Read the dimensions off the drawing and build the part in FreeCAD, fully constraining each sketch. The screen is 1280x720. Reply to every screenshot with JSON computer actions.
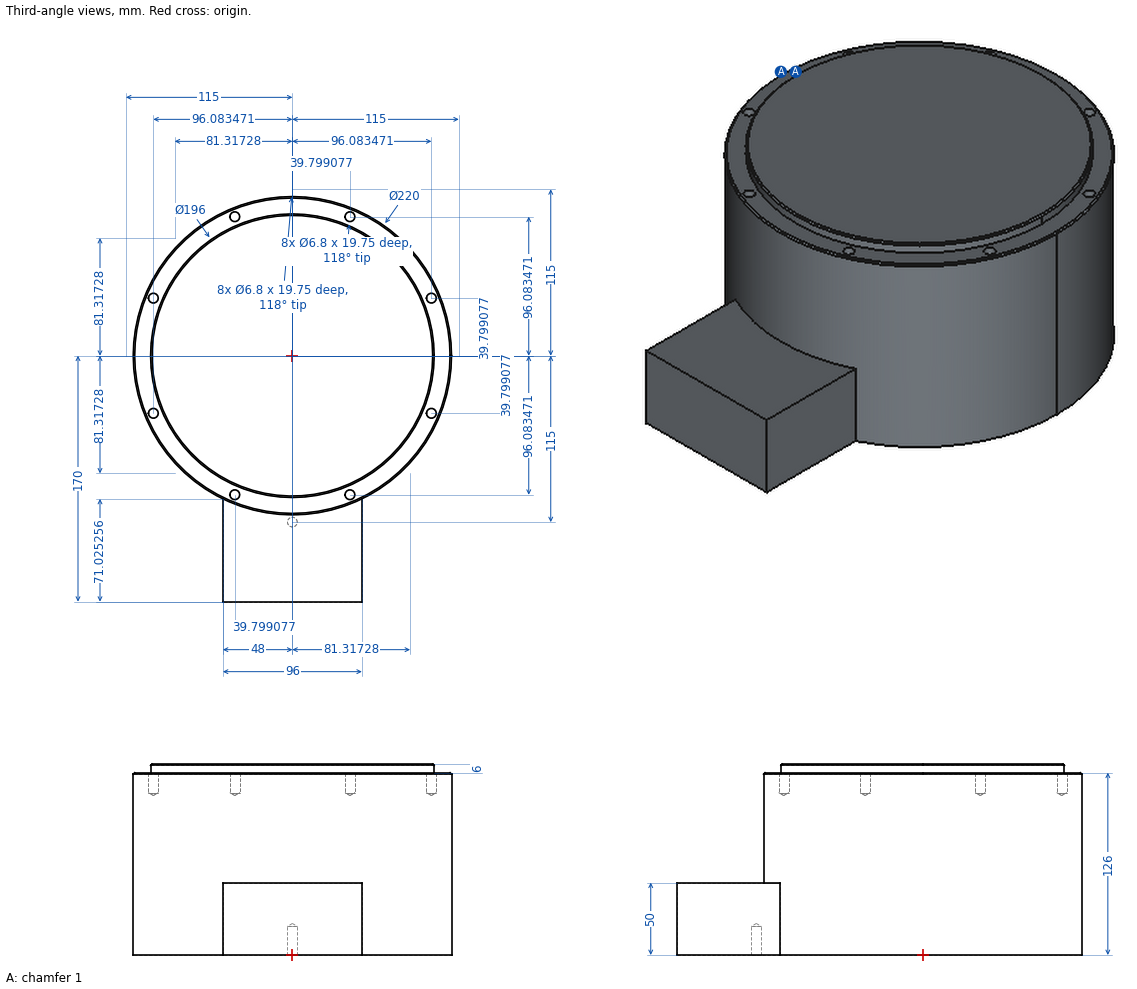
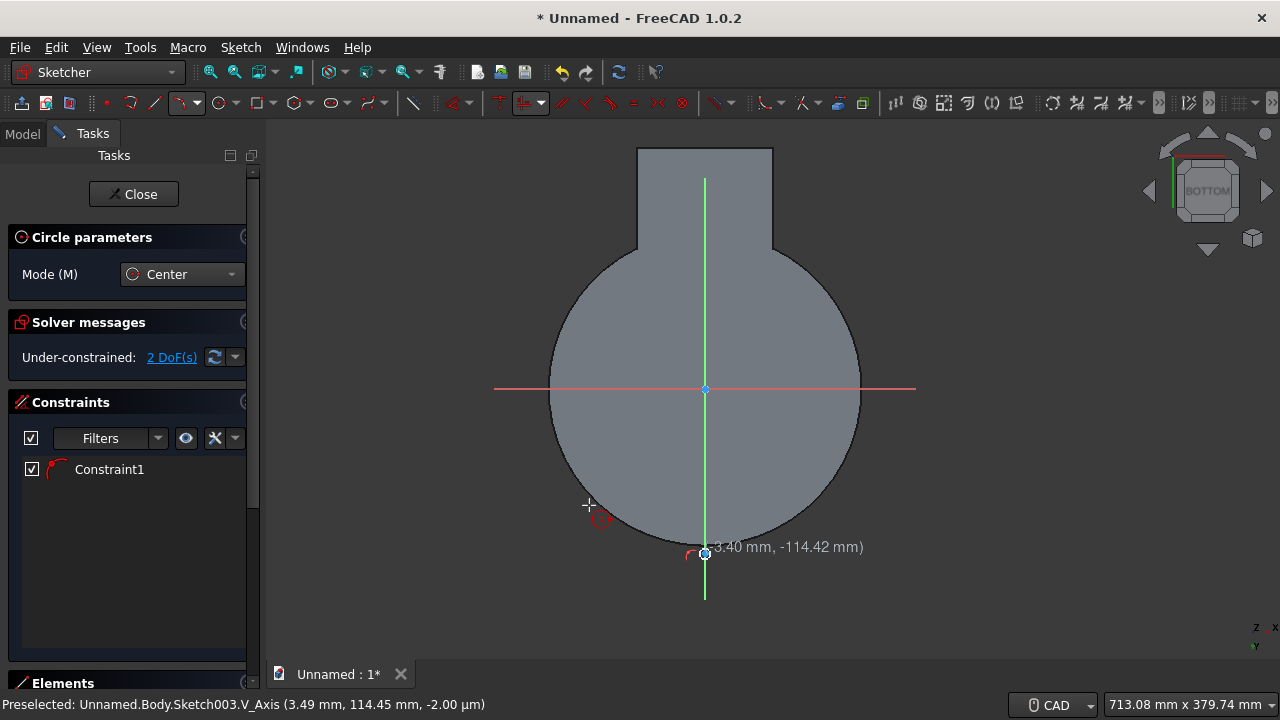
{"action": "left_click", "coordinate": [589, 505]}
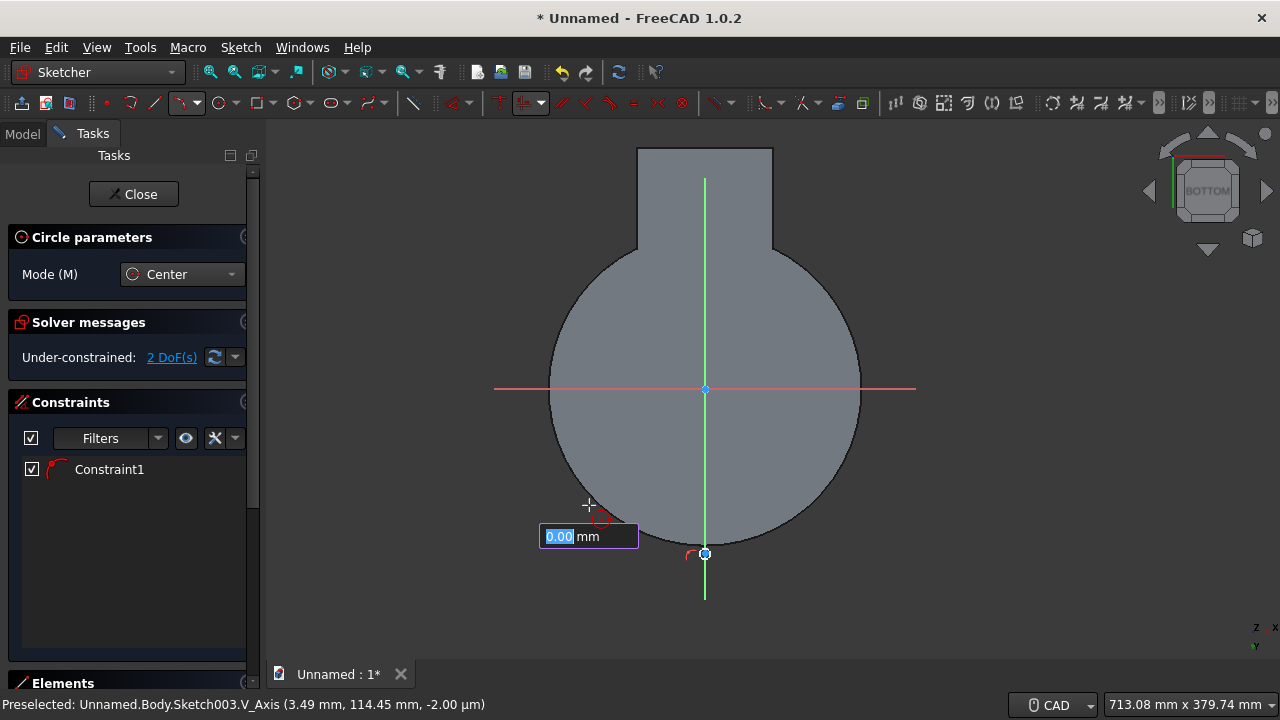
{"action": "scroll", "coordinate": [593, 502], "scroll_direction": "up", "scroll_amount": 6}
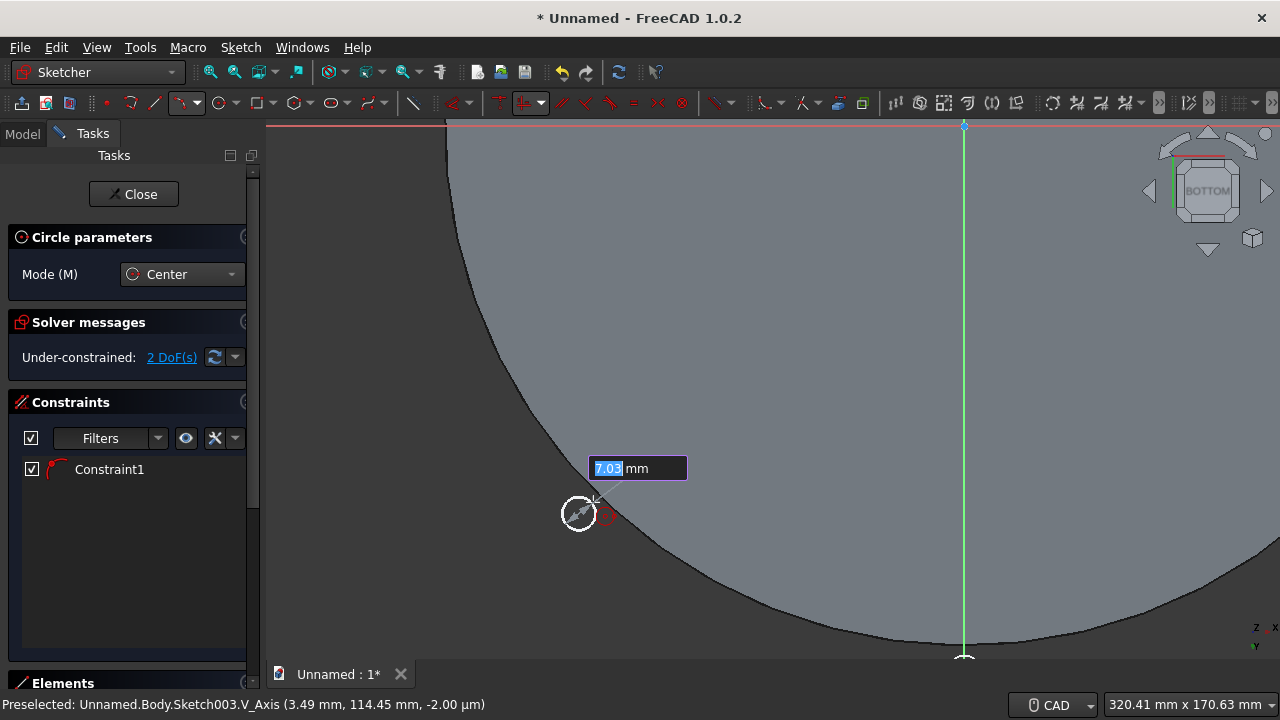
{"action": "left_click", "coordinate": [592, 499]}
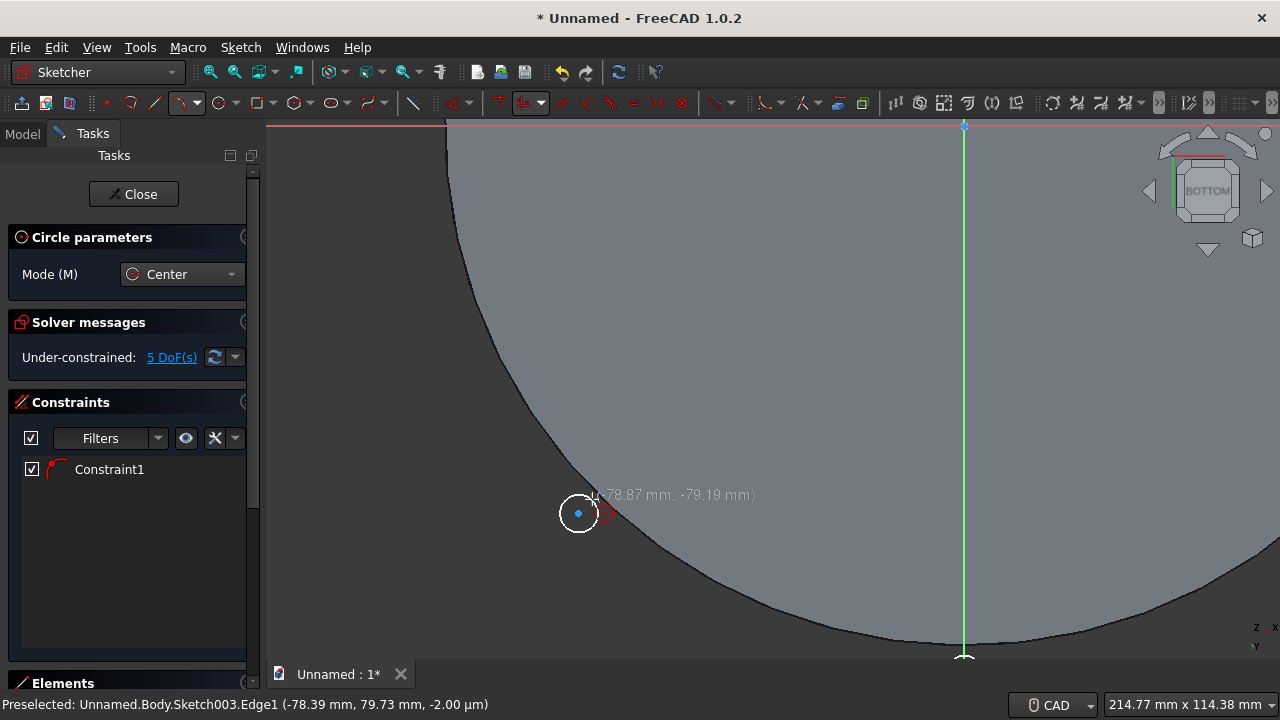
{"action": "scroll", "coordinate": [593, 502], "scroll_direction": "down", "scroll_amount": 6}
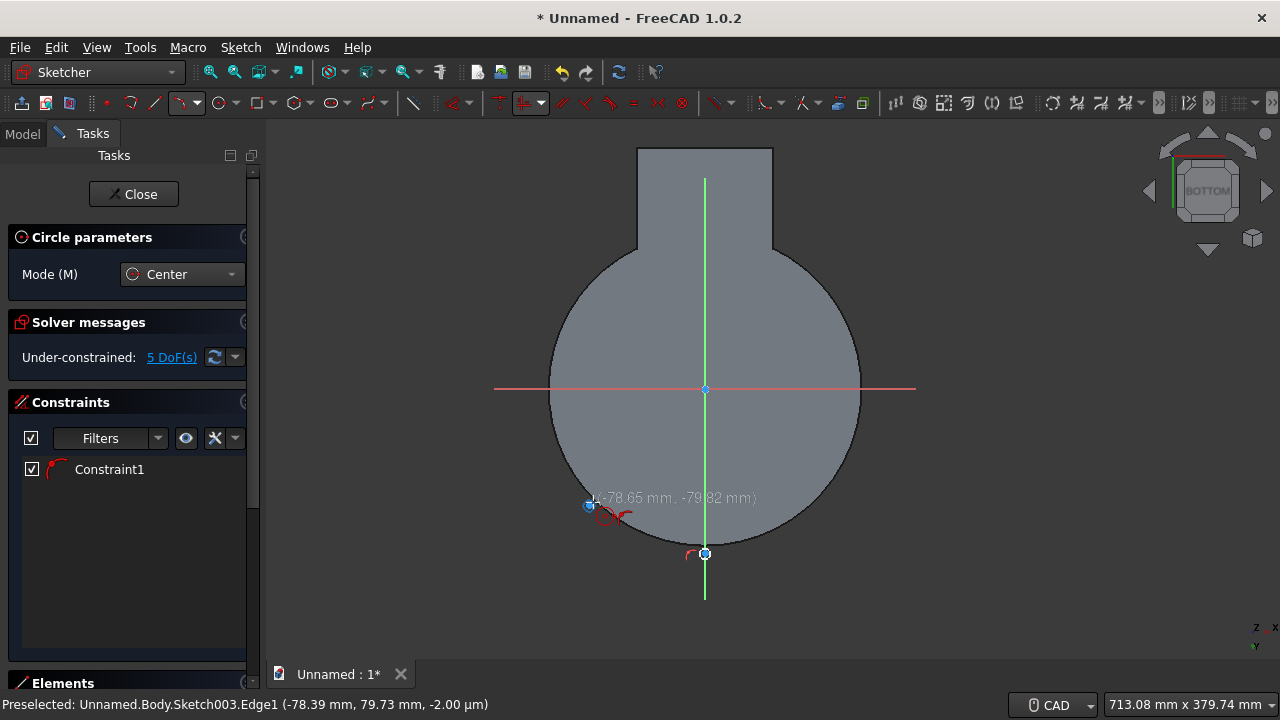
{"action": "scroll", "coordinate": [542, 389], "scroll_direction": "up", "scroll_amount": 8}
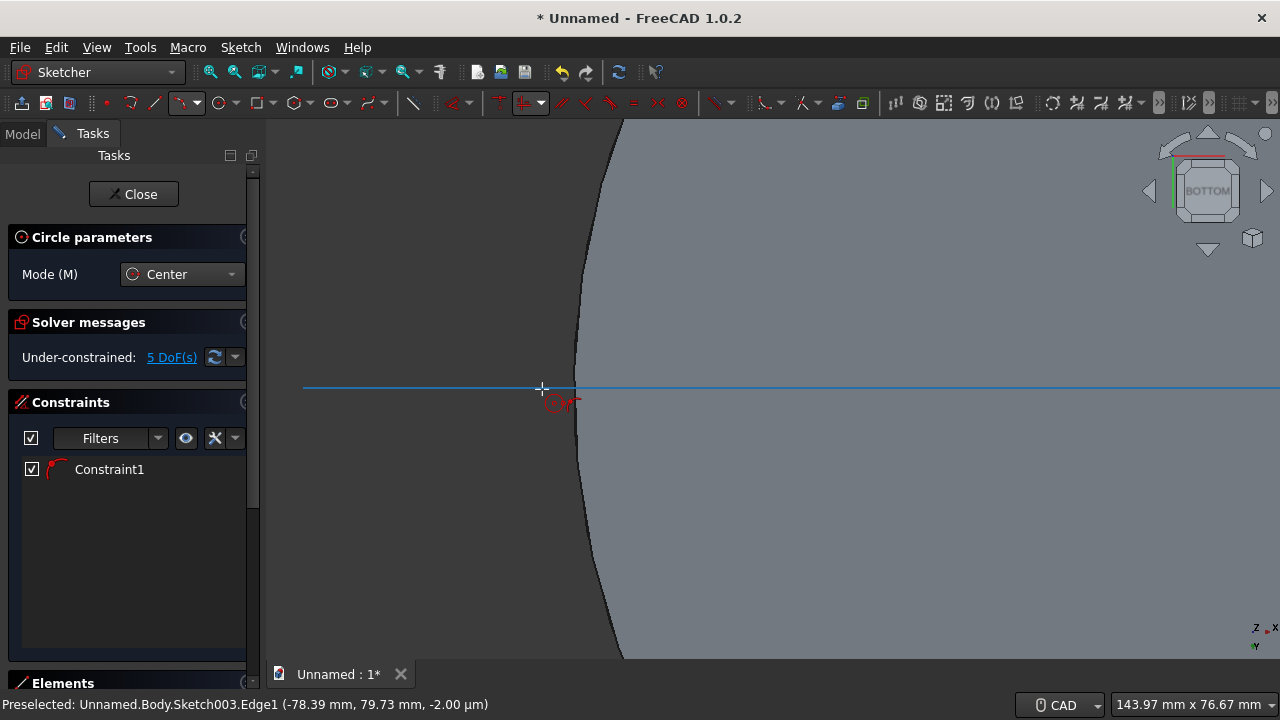
{"action": "scroll", "coordinate": [542, 389], "scroll_direction": "down", "scroll_amount": 8}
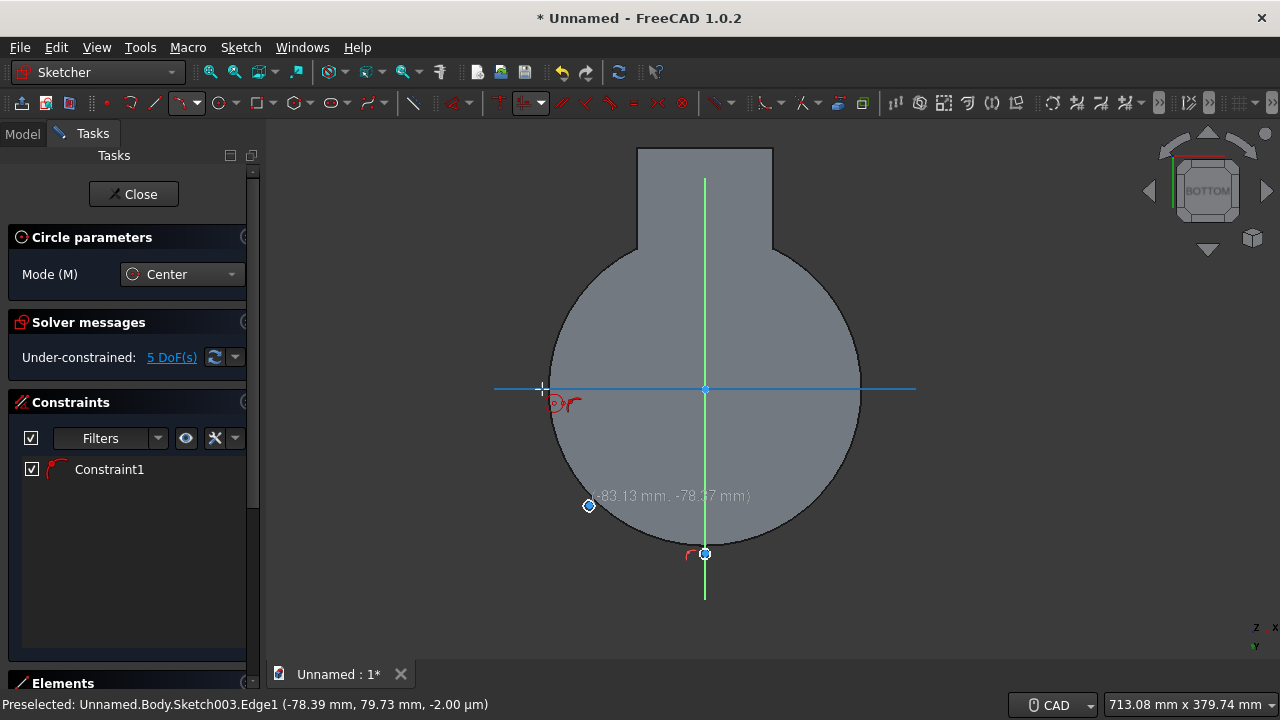
{"action": "left_click", "coordinate": [542, 389]}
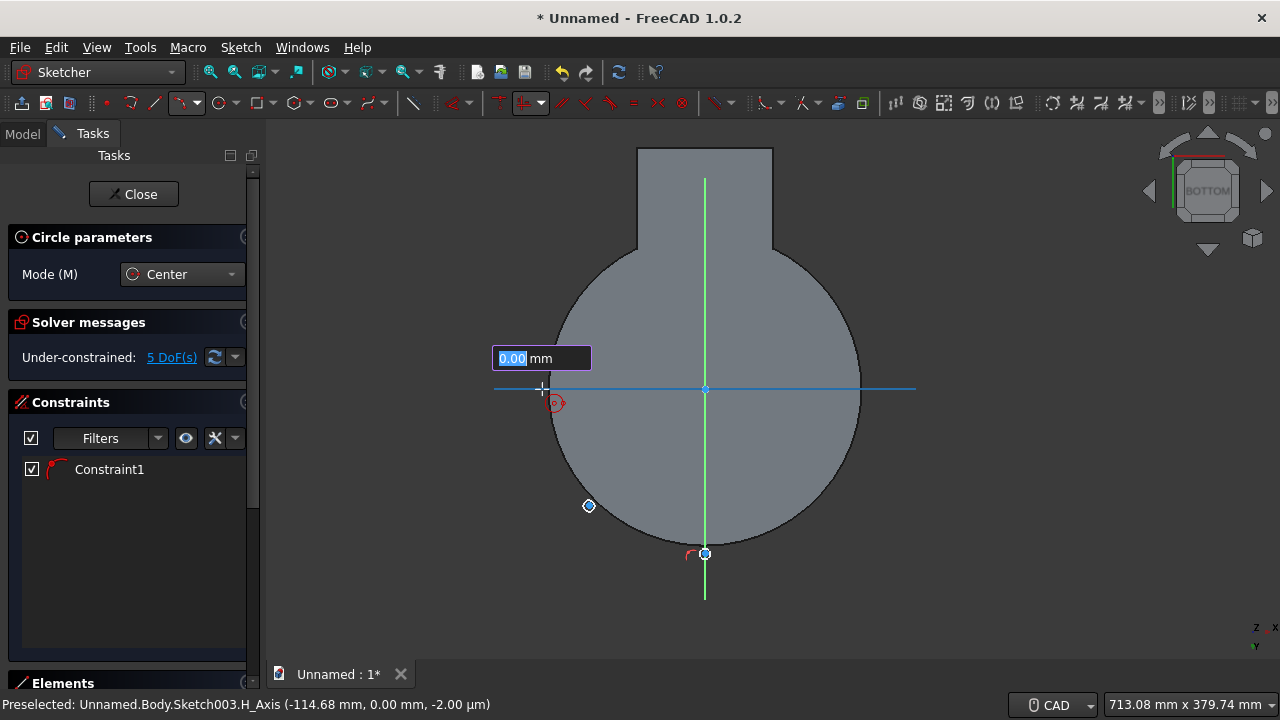
{"action": "scroll", "coordinate": [540, 394], "scroll_direction": "up", "scroll_amount": 7}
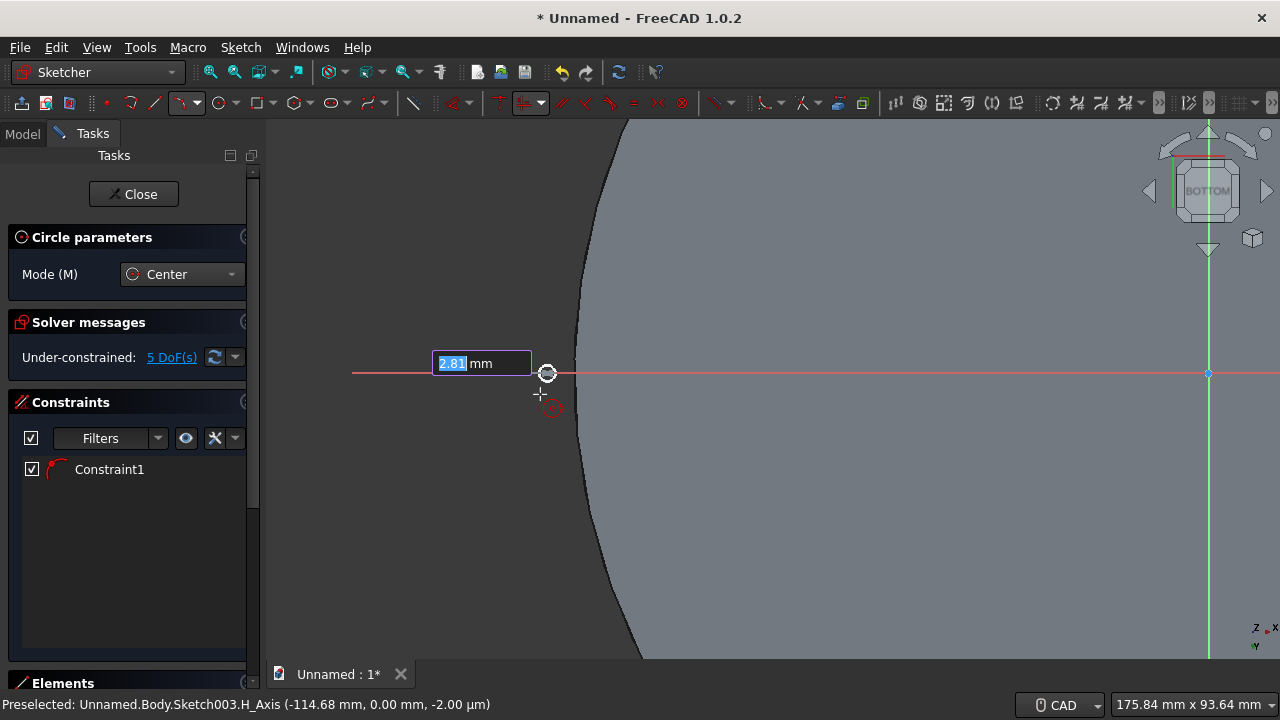
{"action": "left_click", "coordinate": [539, 392]}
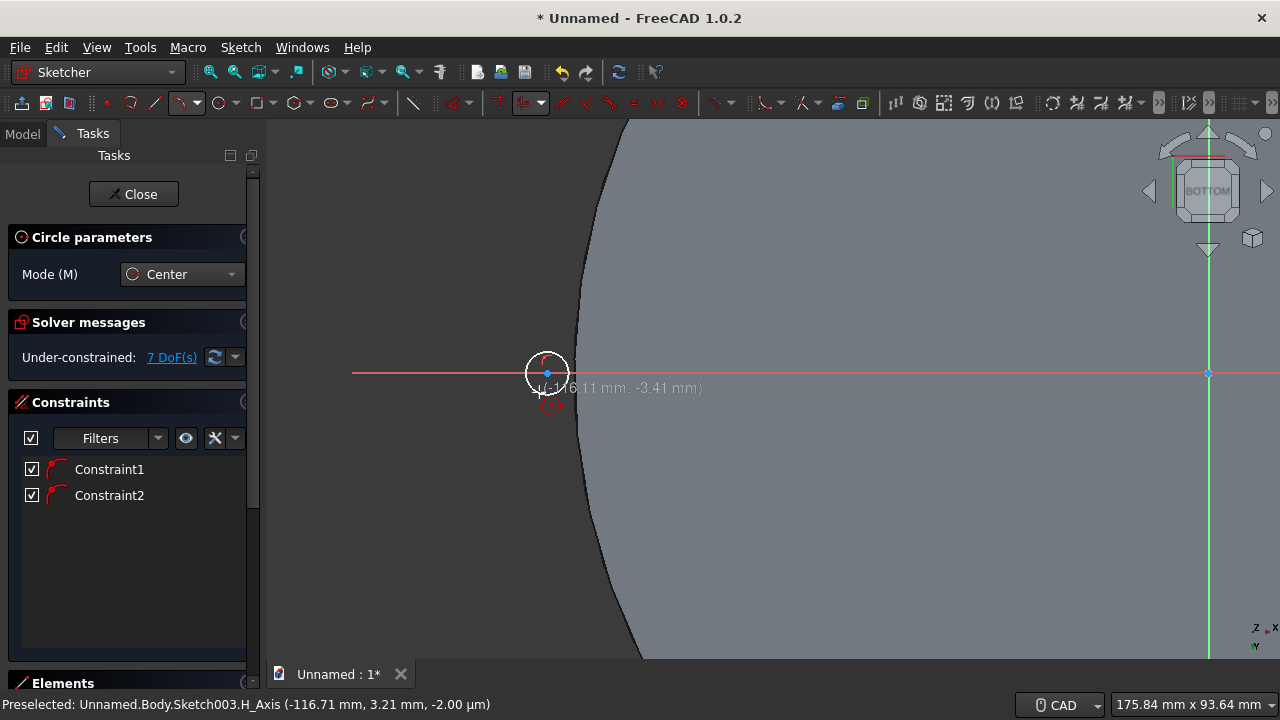
{"action": "scroll", "coordinate": [540, 394], "scroll_direction": "down", "scroll_amount": 7}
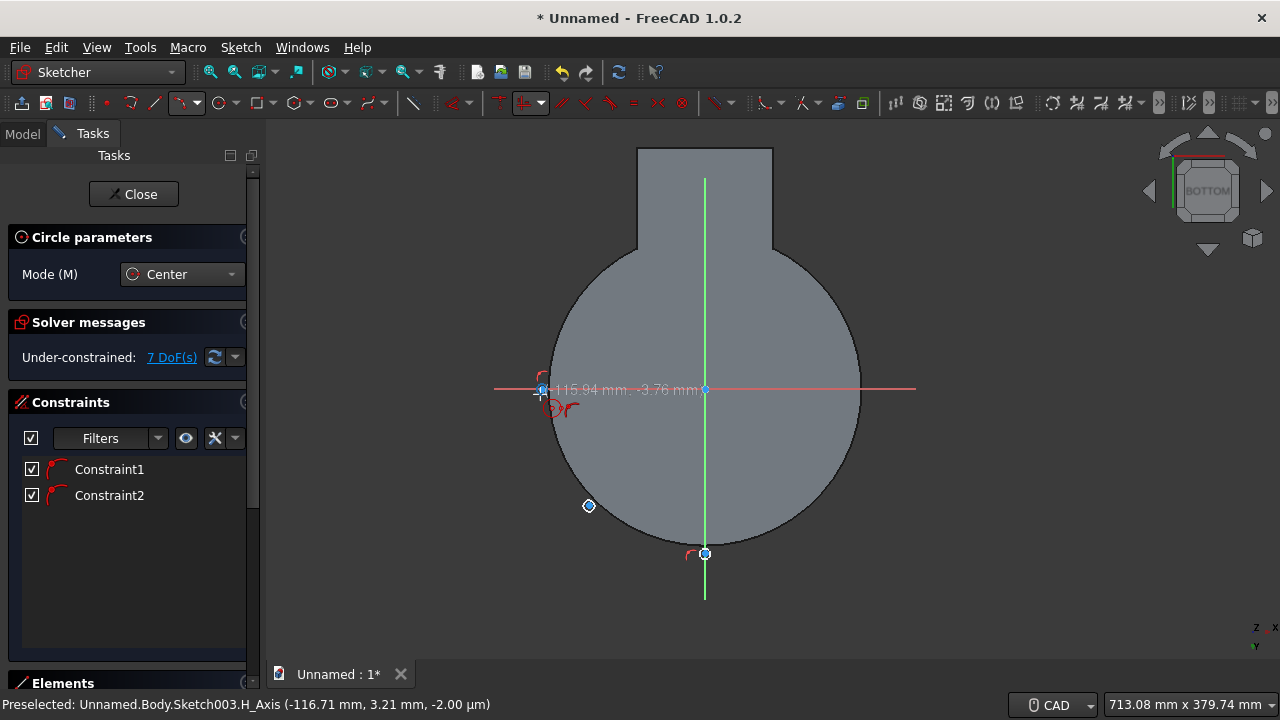
{"action": "scroll", "coordinate": [589, 274], "scroll_direction": "up", "scroll_amount": 8}